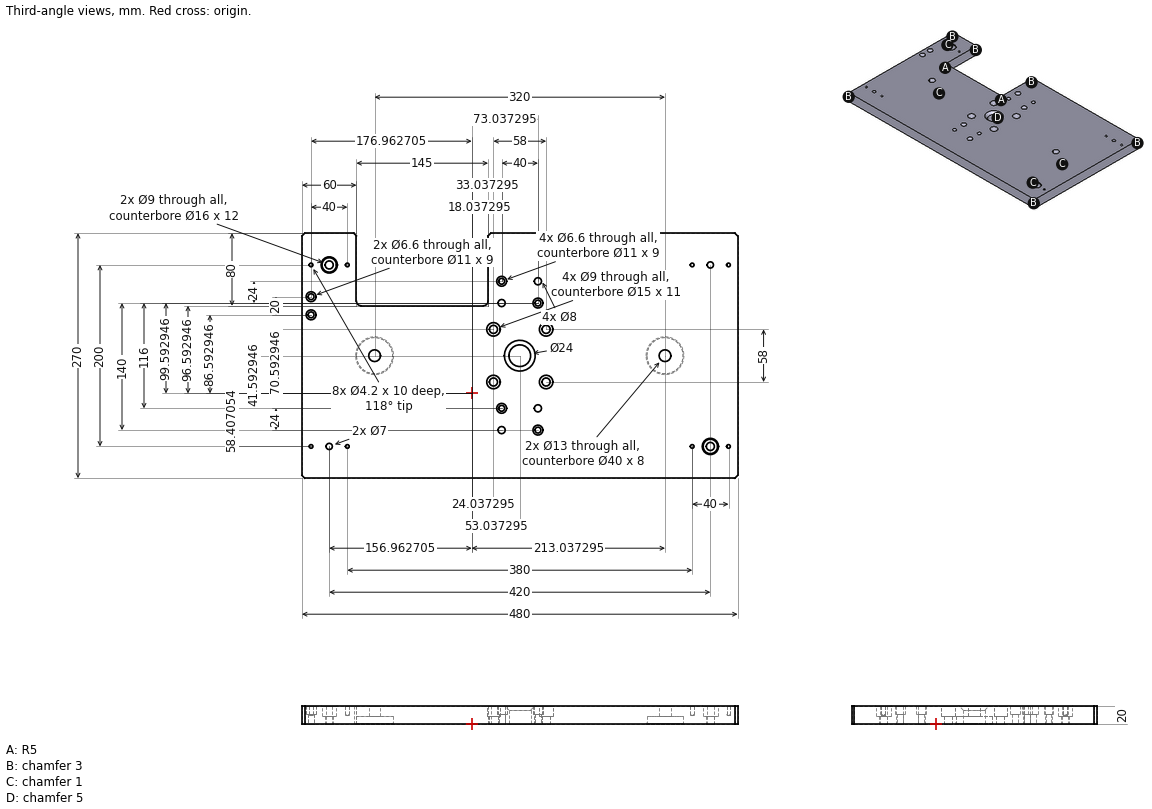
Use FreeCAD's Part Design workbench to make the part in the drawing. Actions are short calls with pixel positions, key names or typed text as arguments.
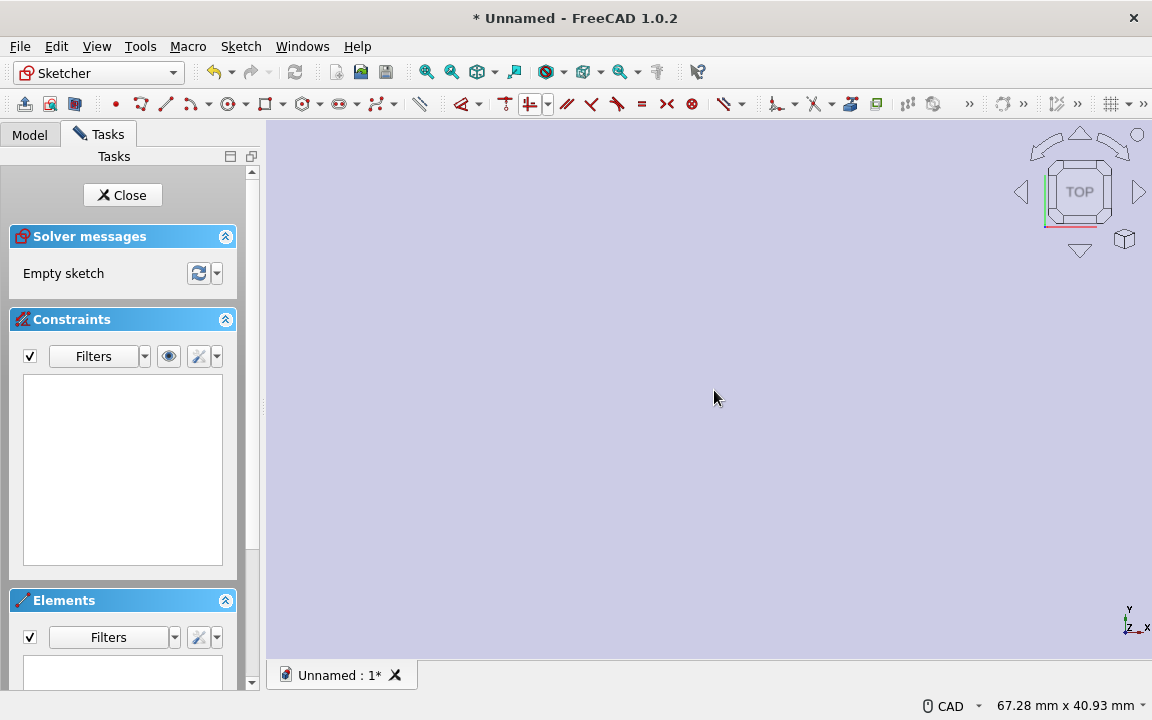
click(228, 104)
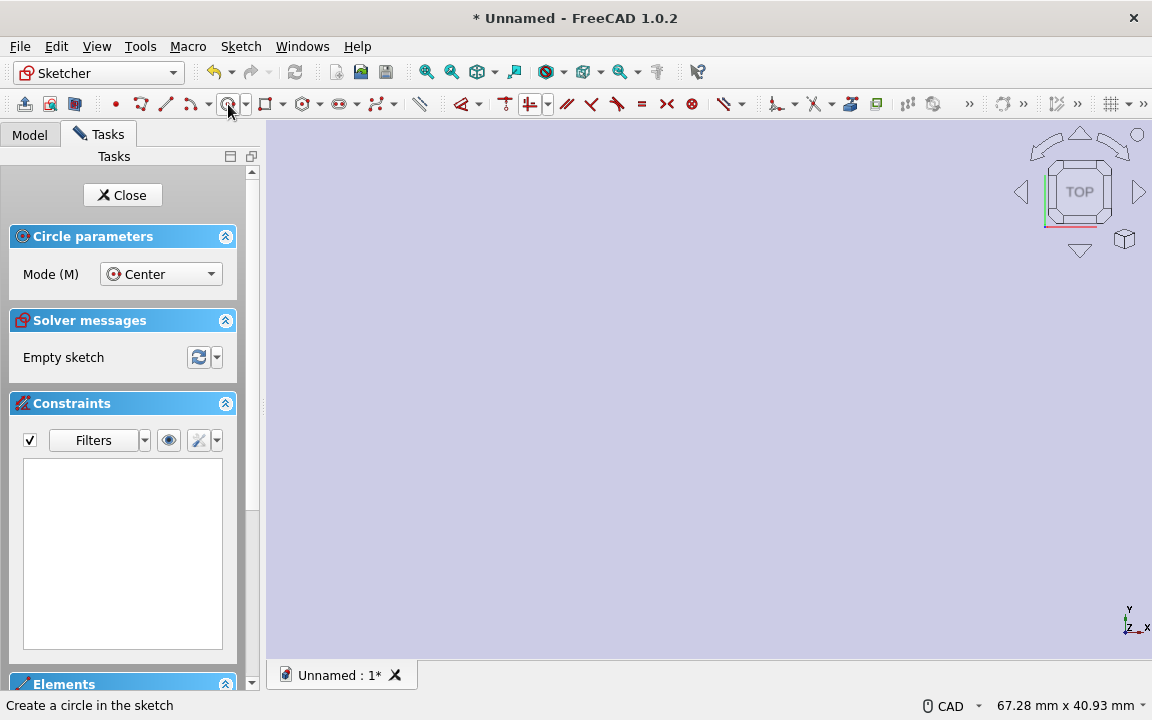
click(640, 377)
click(752, 265)
key(Escape)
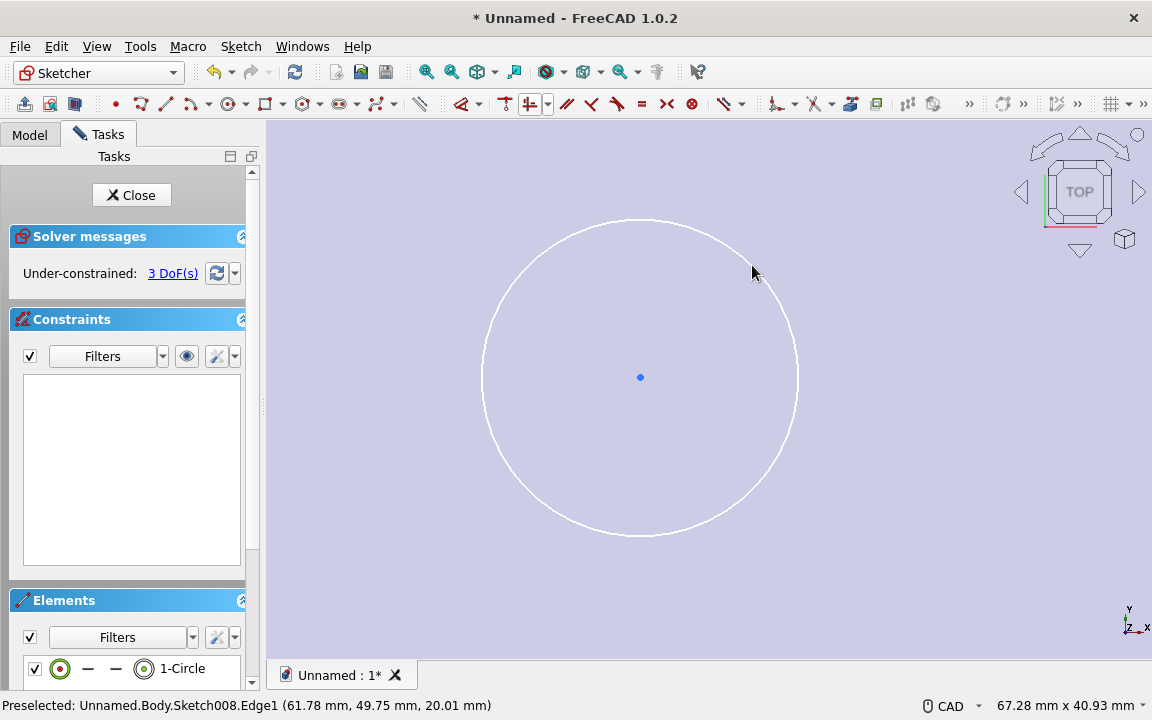
key(d)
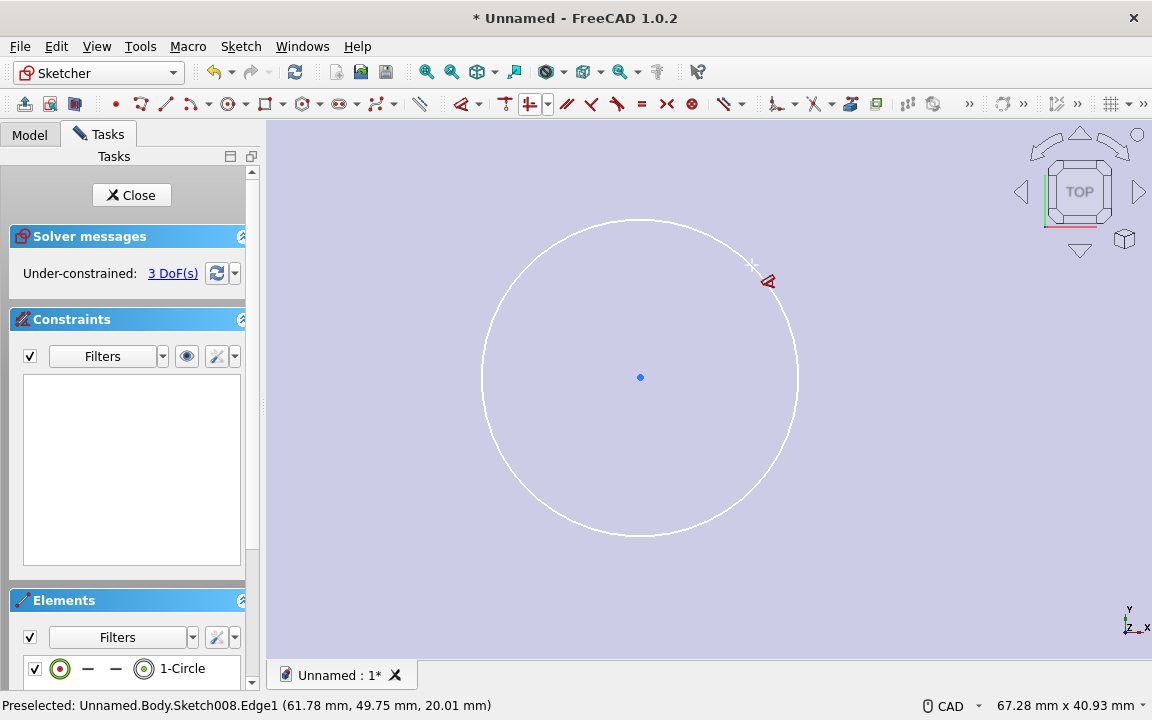
click(752, 266)
click(775, 243)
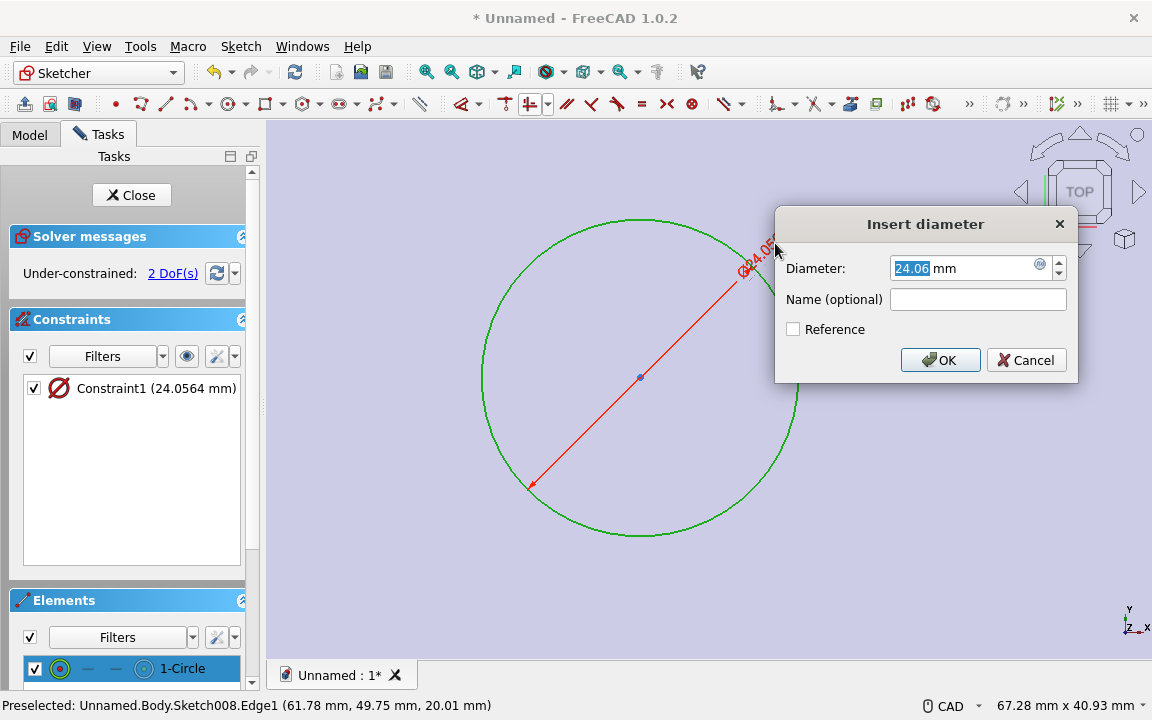
text(24)
key(Return)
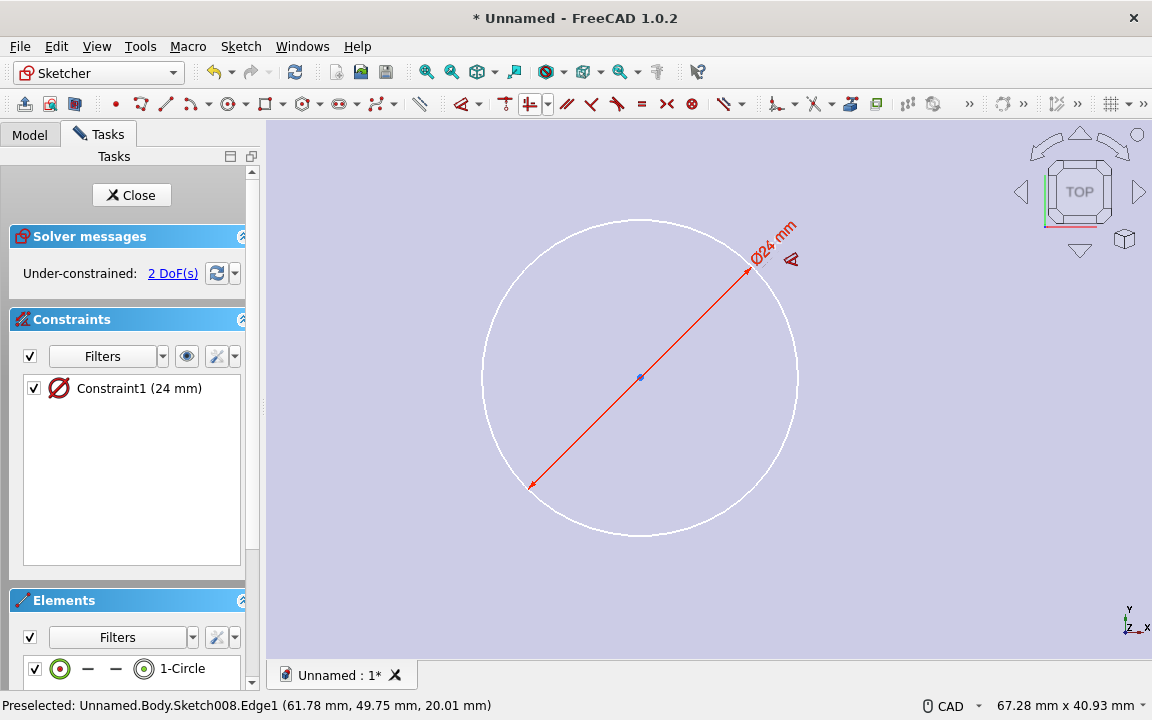
click(640, 378)
click(467, 344)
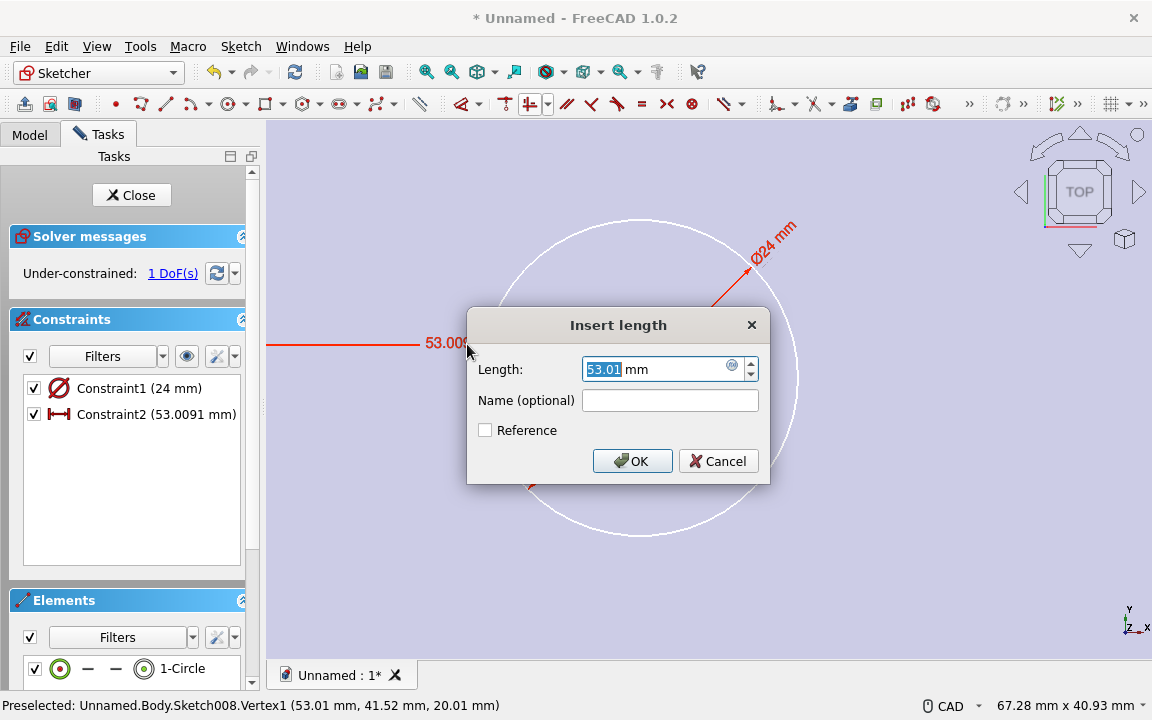
text(53.037295)
key(Return)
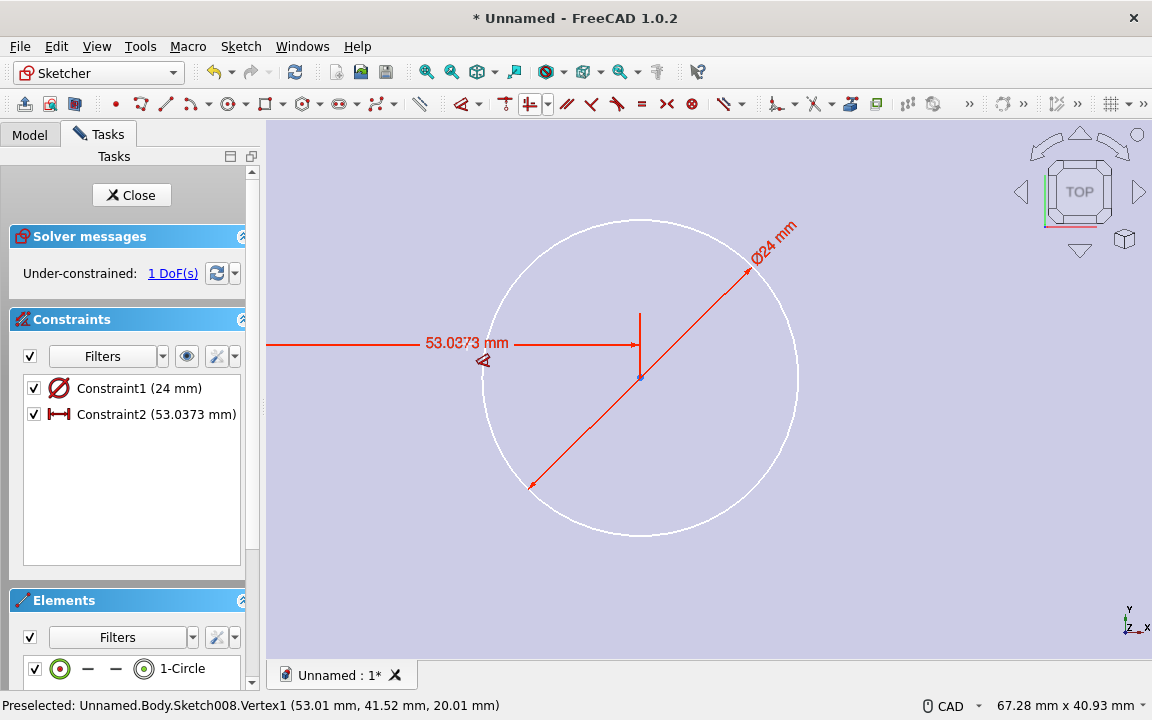
click(640, 378)
click(674, 505)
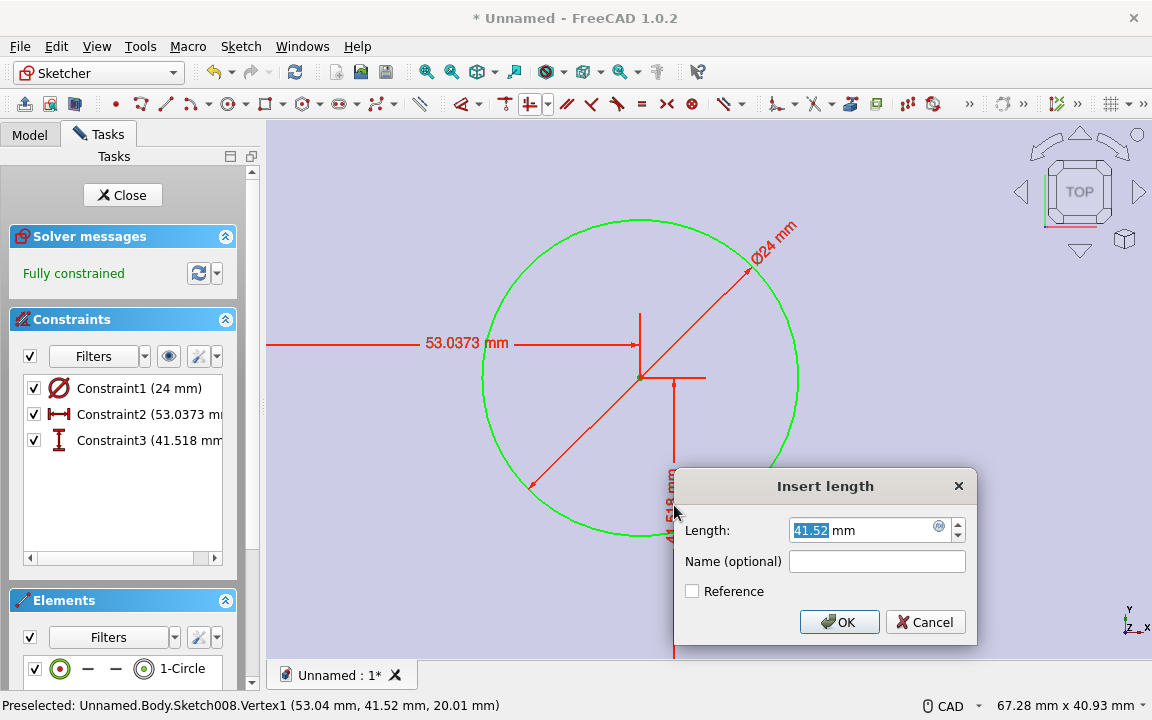
text(41.592946)
key(Return)
key(Escape)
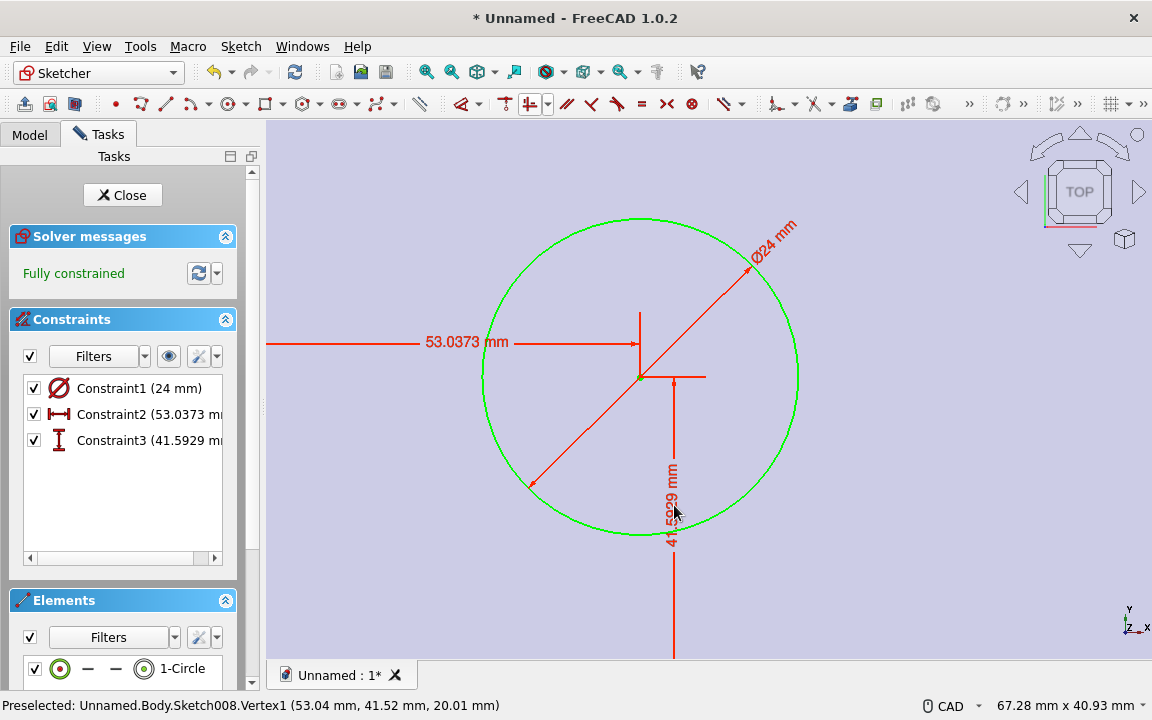
click(123, 195)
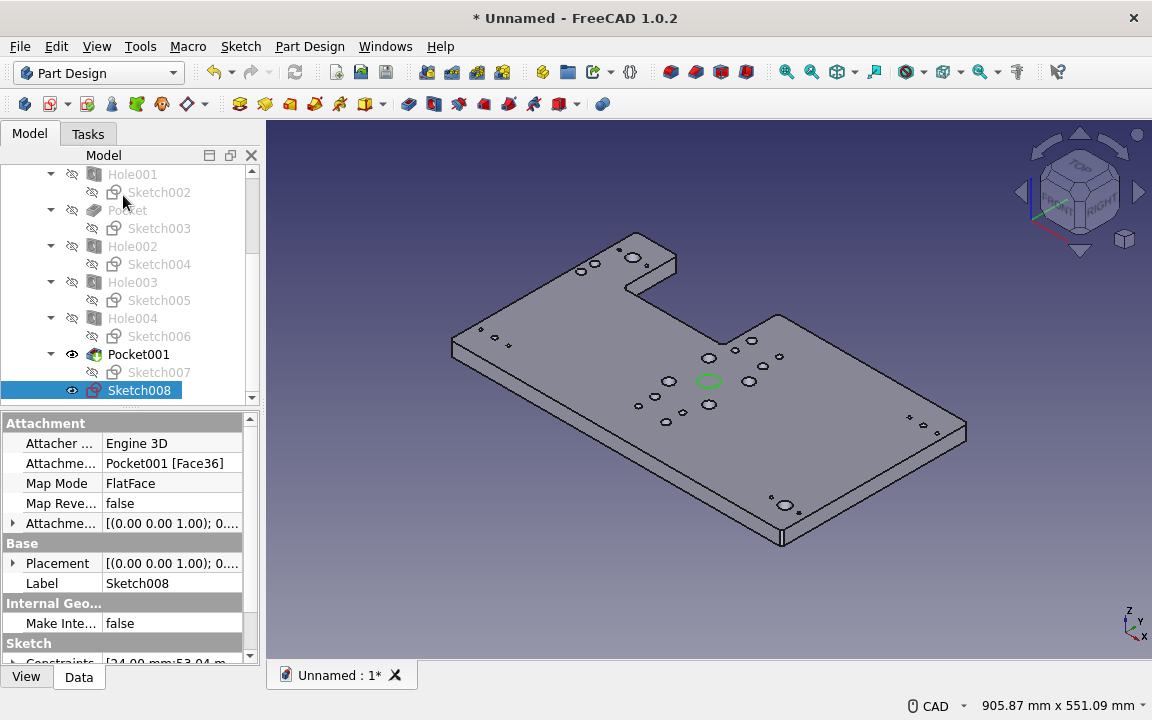
click(409, 104)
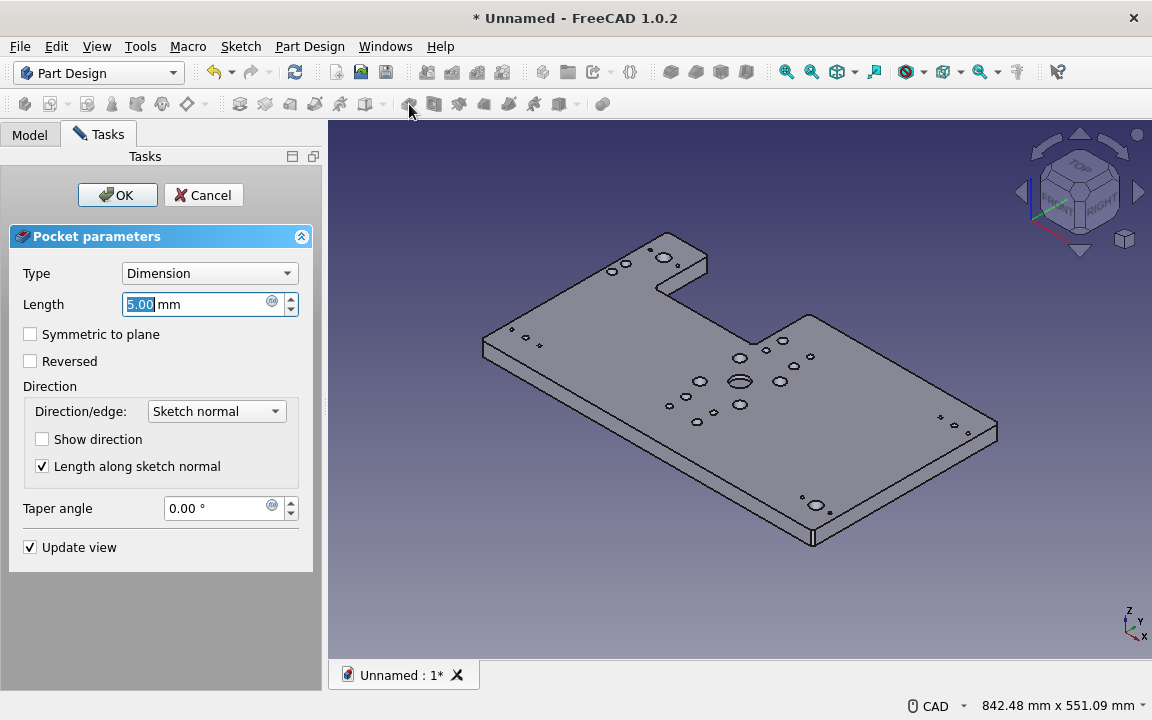
click(210, 274)